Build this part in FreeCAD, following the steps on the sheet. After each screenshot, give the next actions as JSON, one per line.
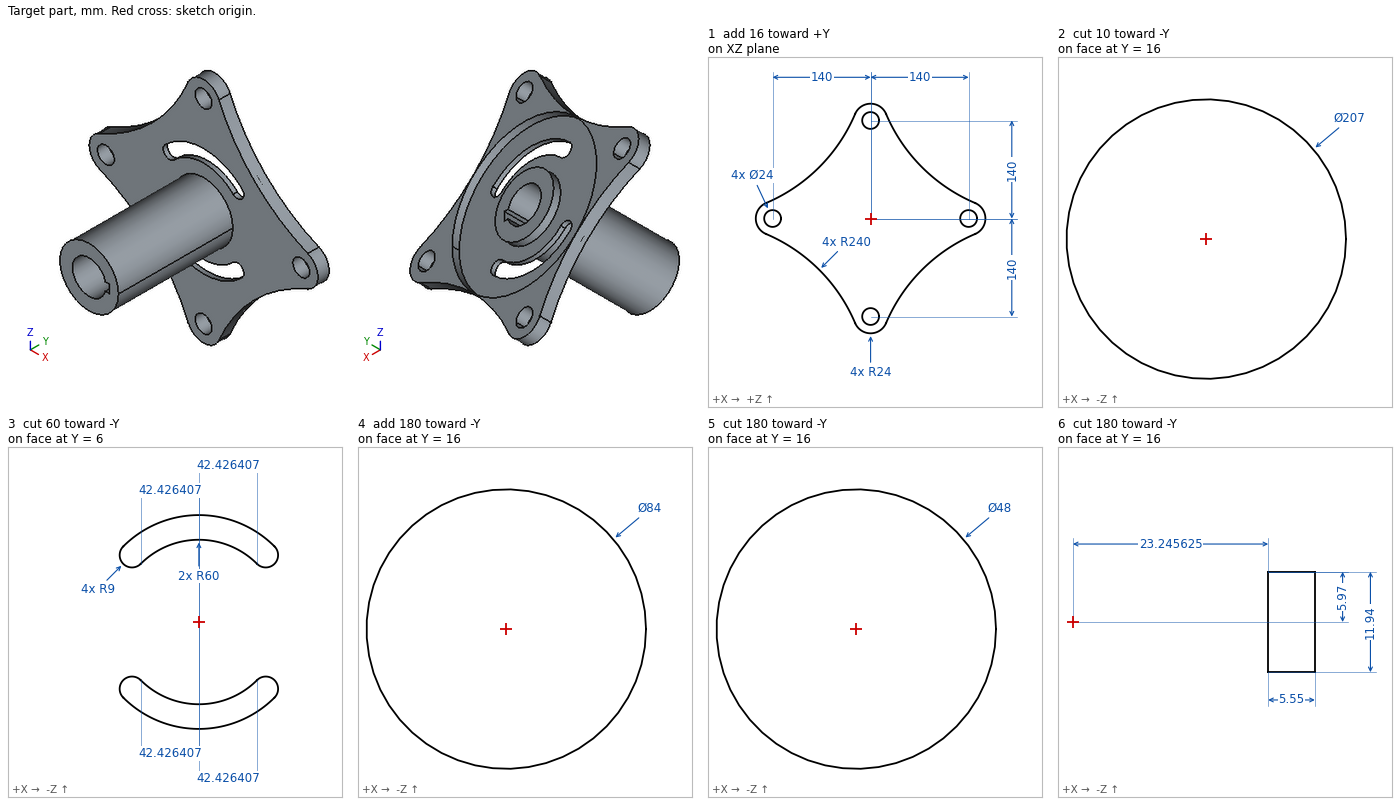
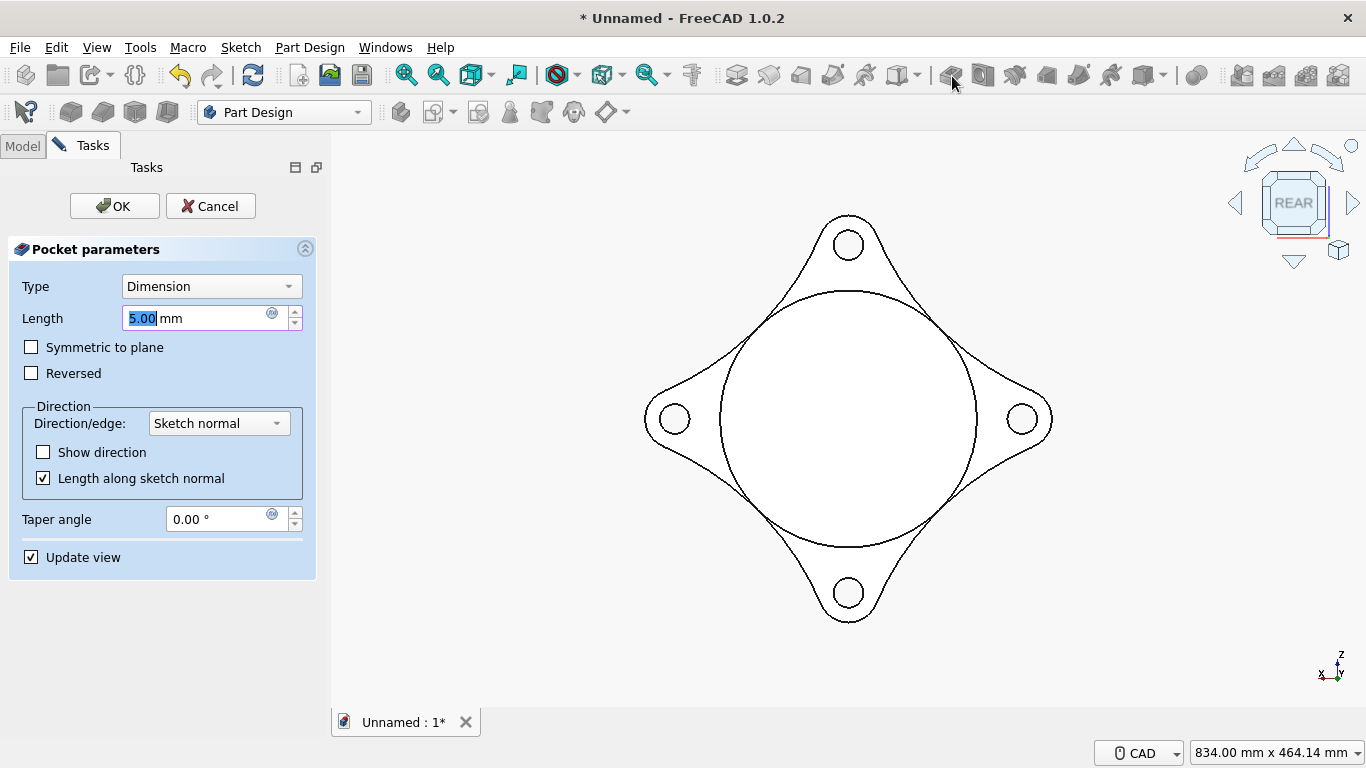
{"action": "type", "text": "10"}
{"action": "key", "text": "Tab"}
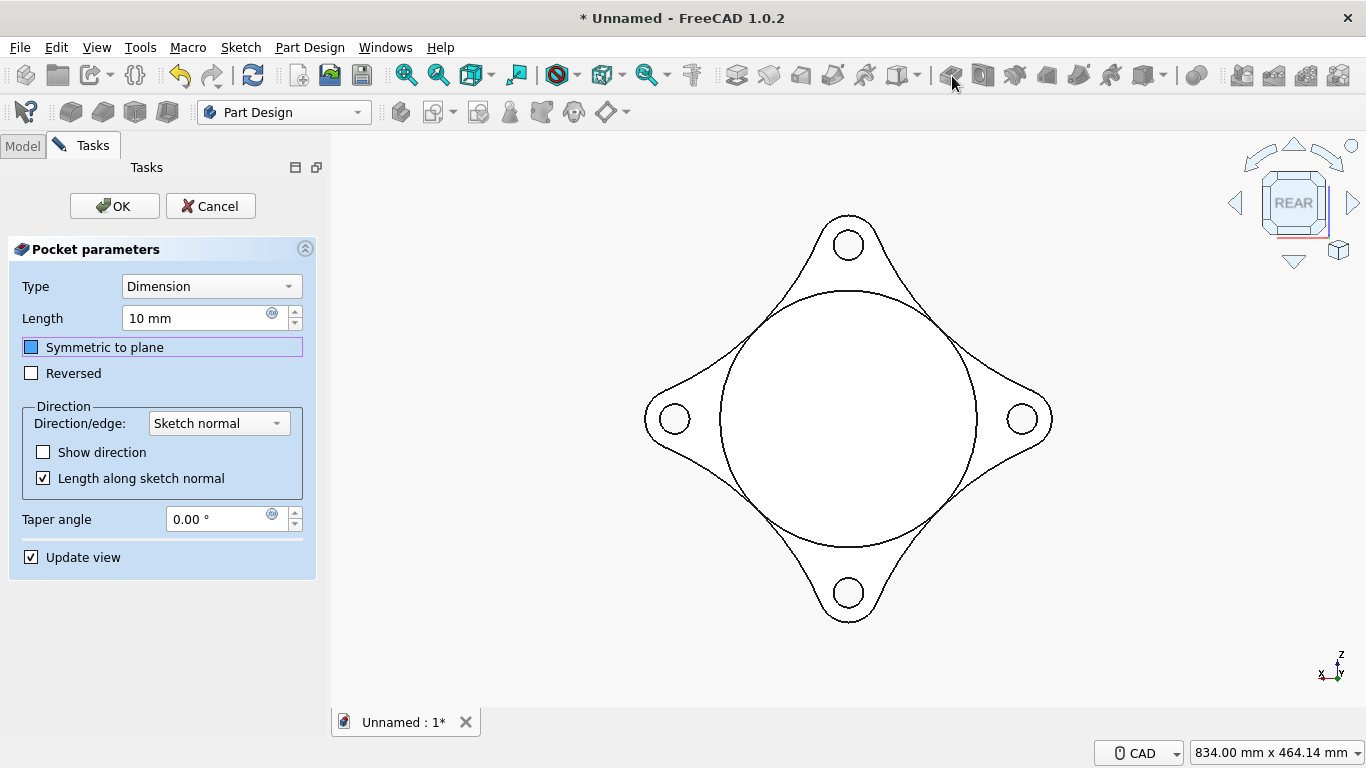
{"action": "left_click", "coordinate": [115, 206]}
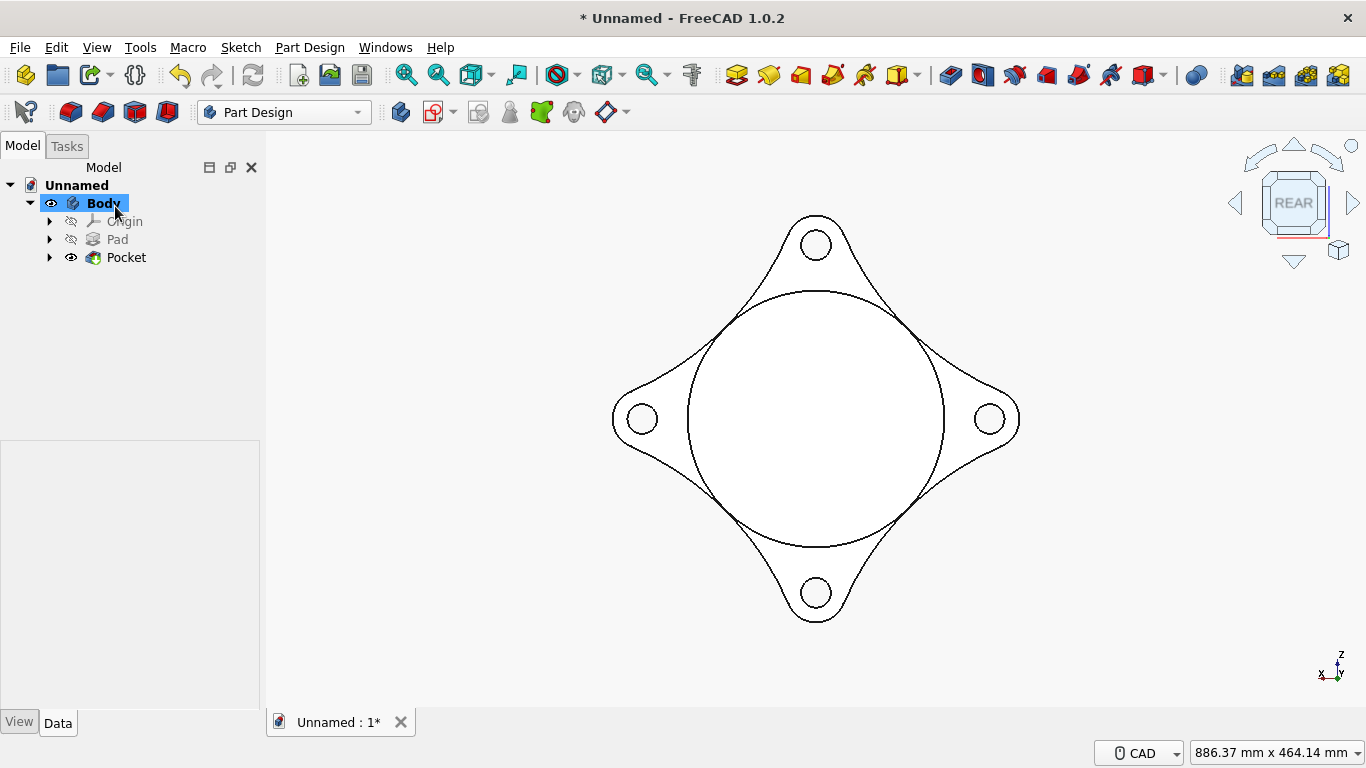
{"action": "left_click", "coordinate": [816, 418]}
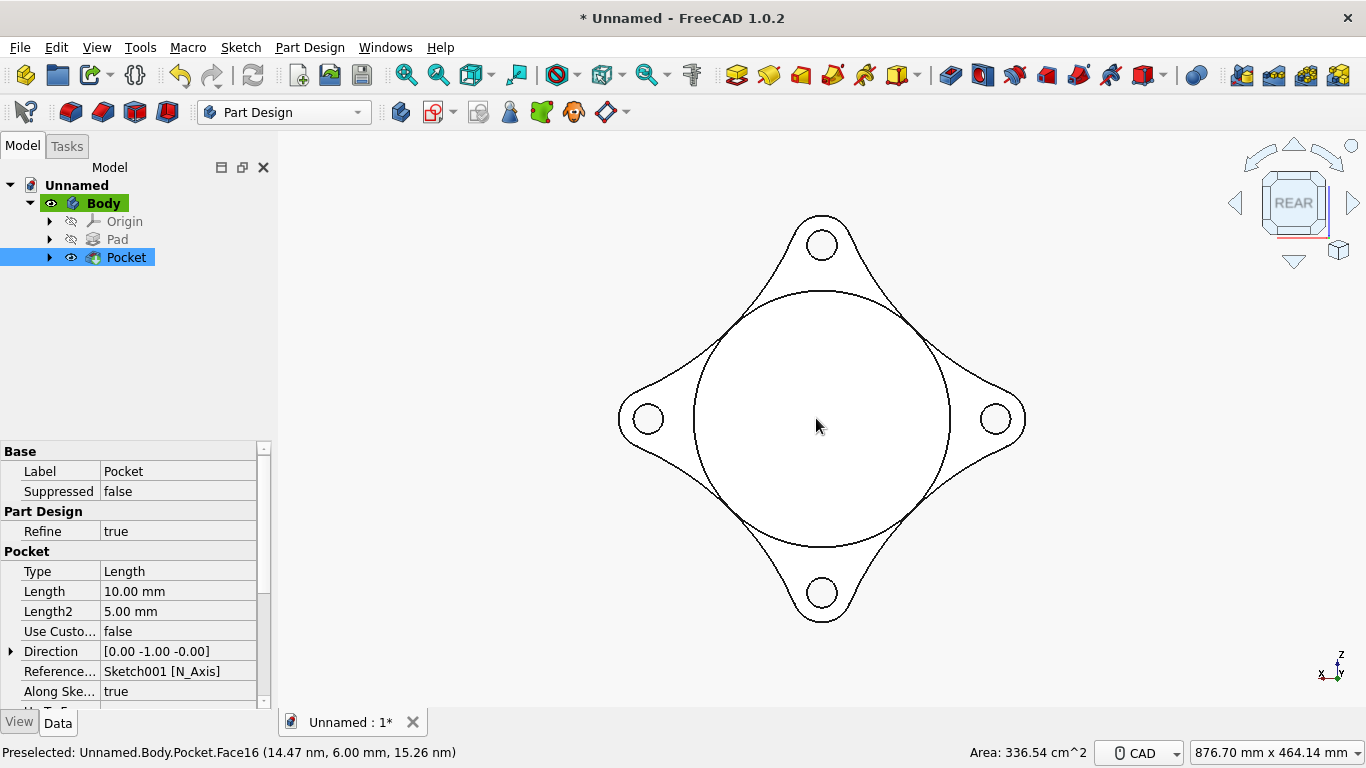
{"action": "left_click", "coordinate": [434, 112]}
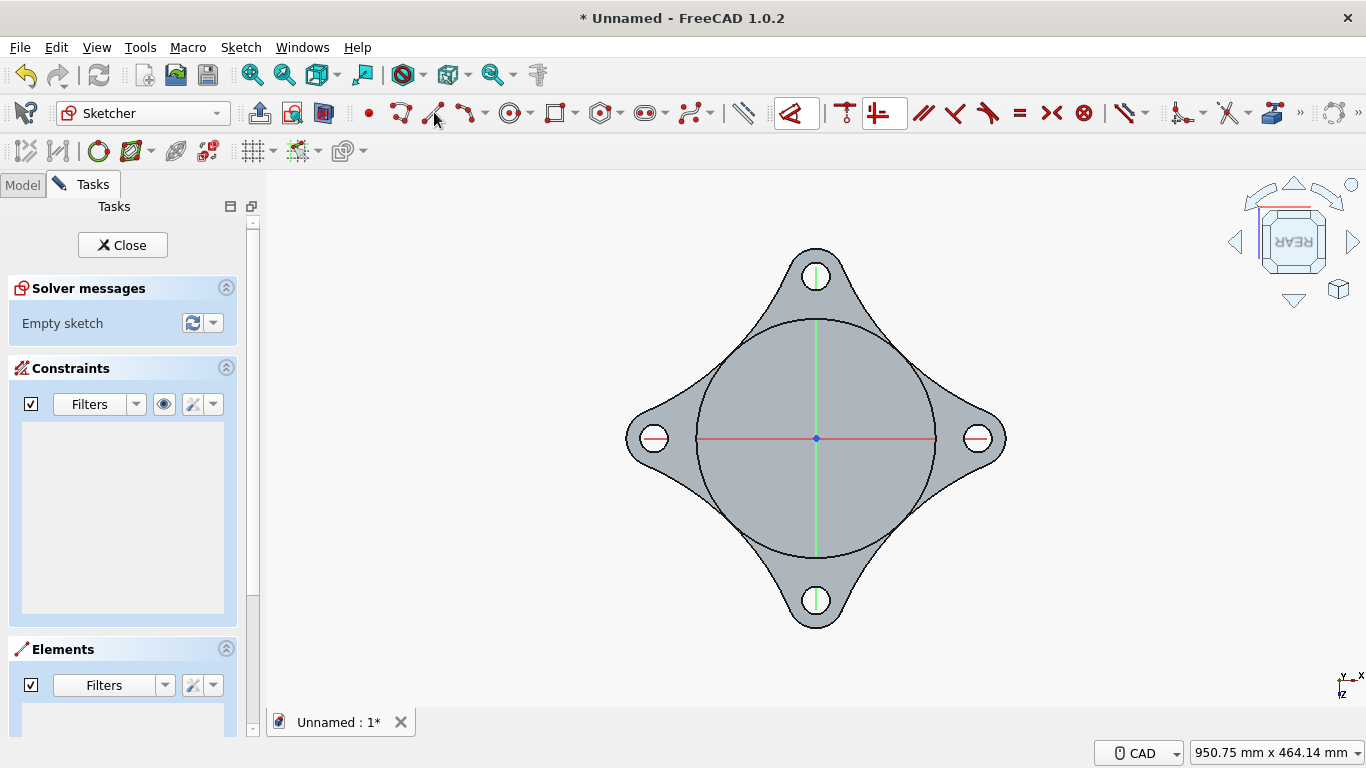
{"action": "left_click", "coordinate": [324, 114]}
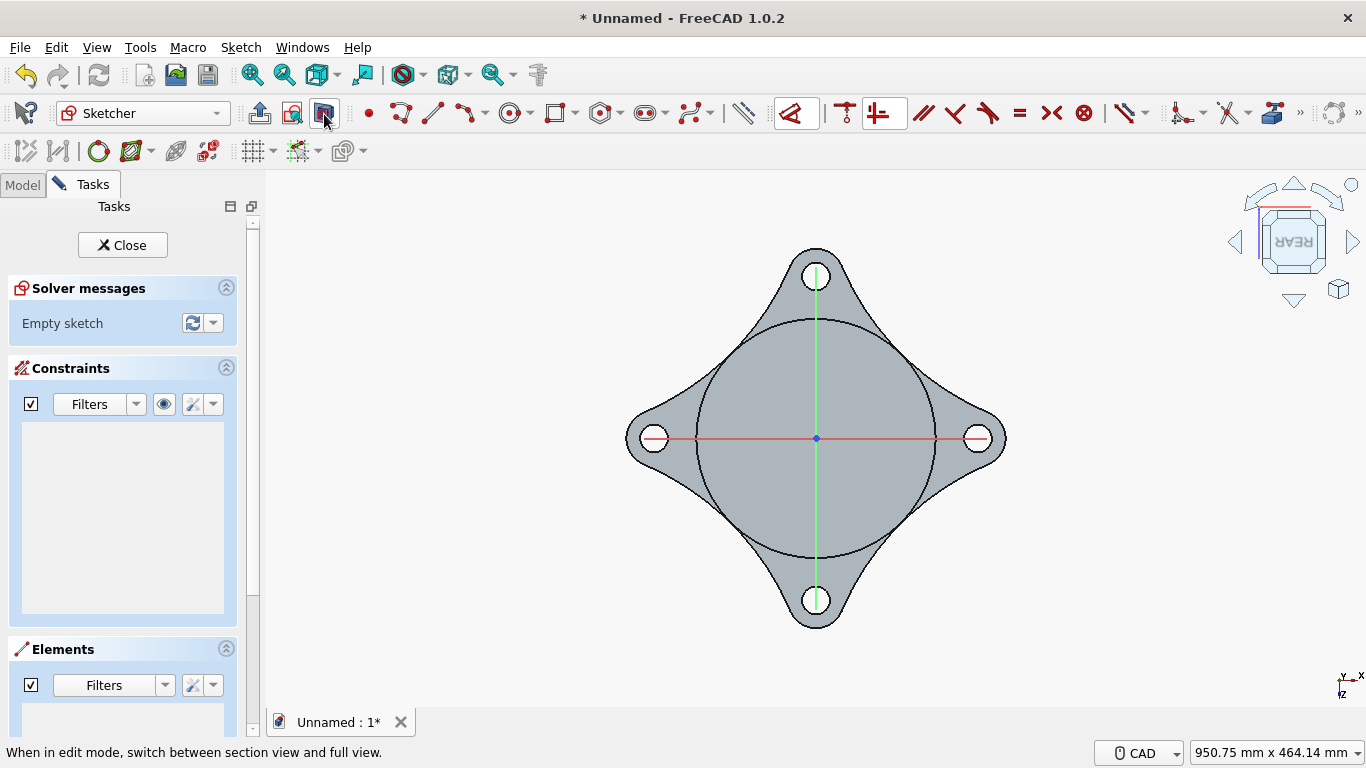
{"action": "scroll", "coordinate": [899, 438], "scroll_direction": "up", "scroll_amount": 3}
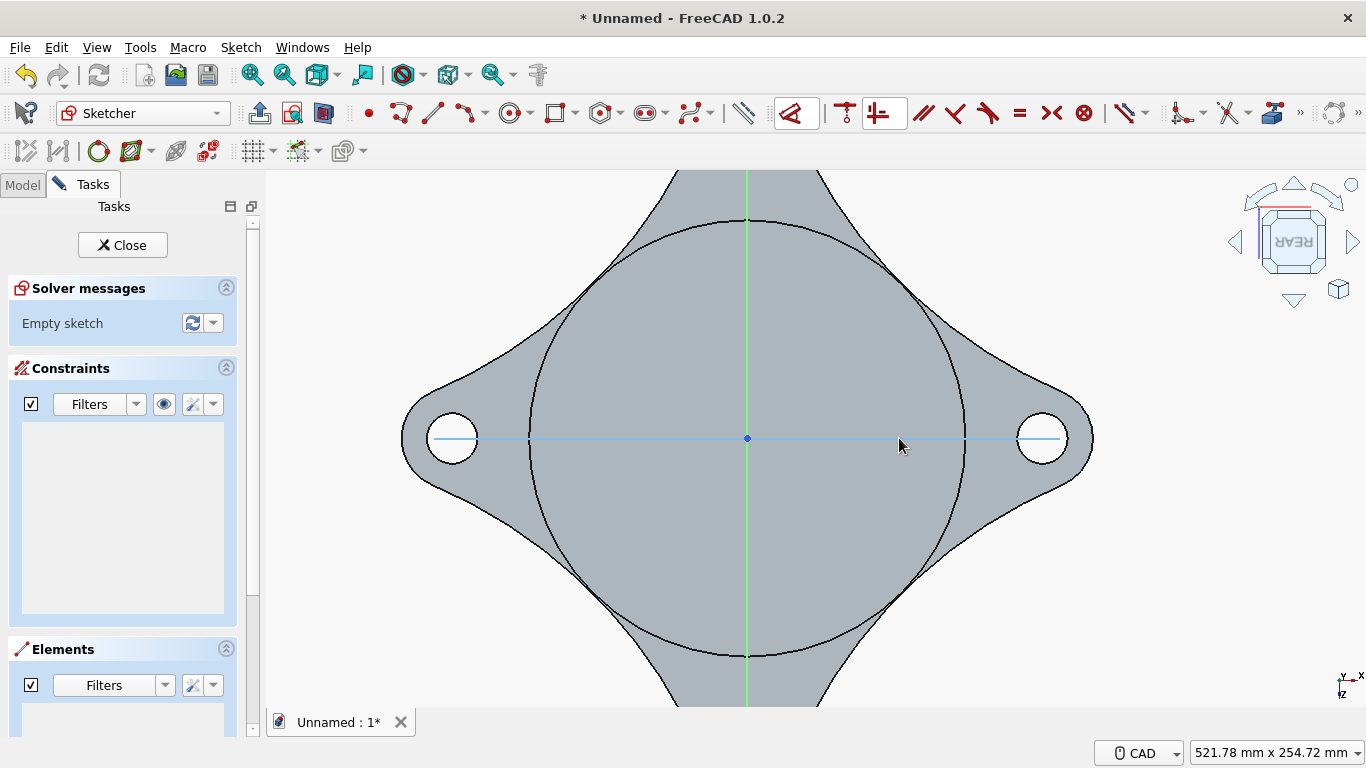
{"action": "left_click", "coordinate": [466, 114]}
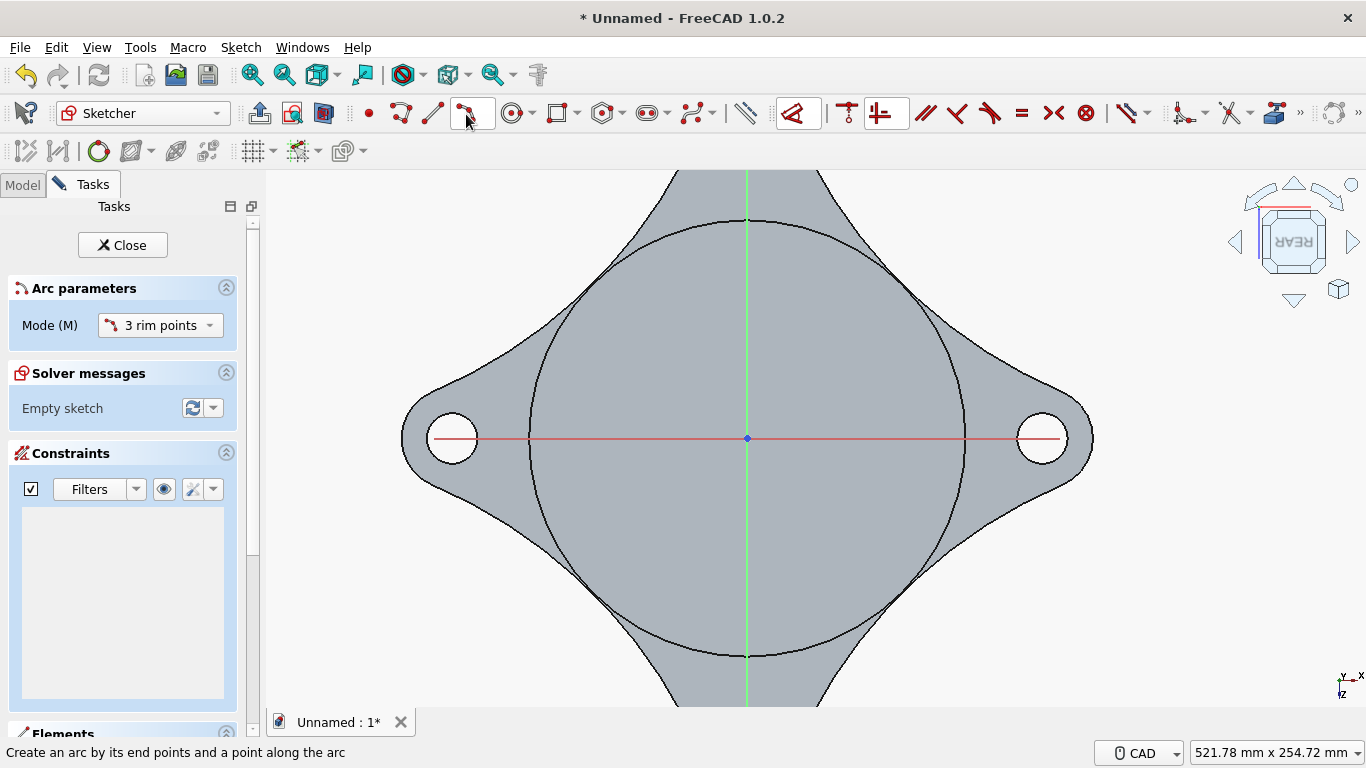
{"action": "left_click", "coordinate": [658, 349]}
{"action": "left_click", "coordinate": [837, 349]}
{"action": "left_click", "coordinate": [767, 314]}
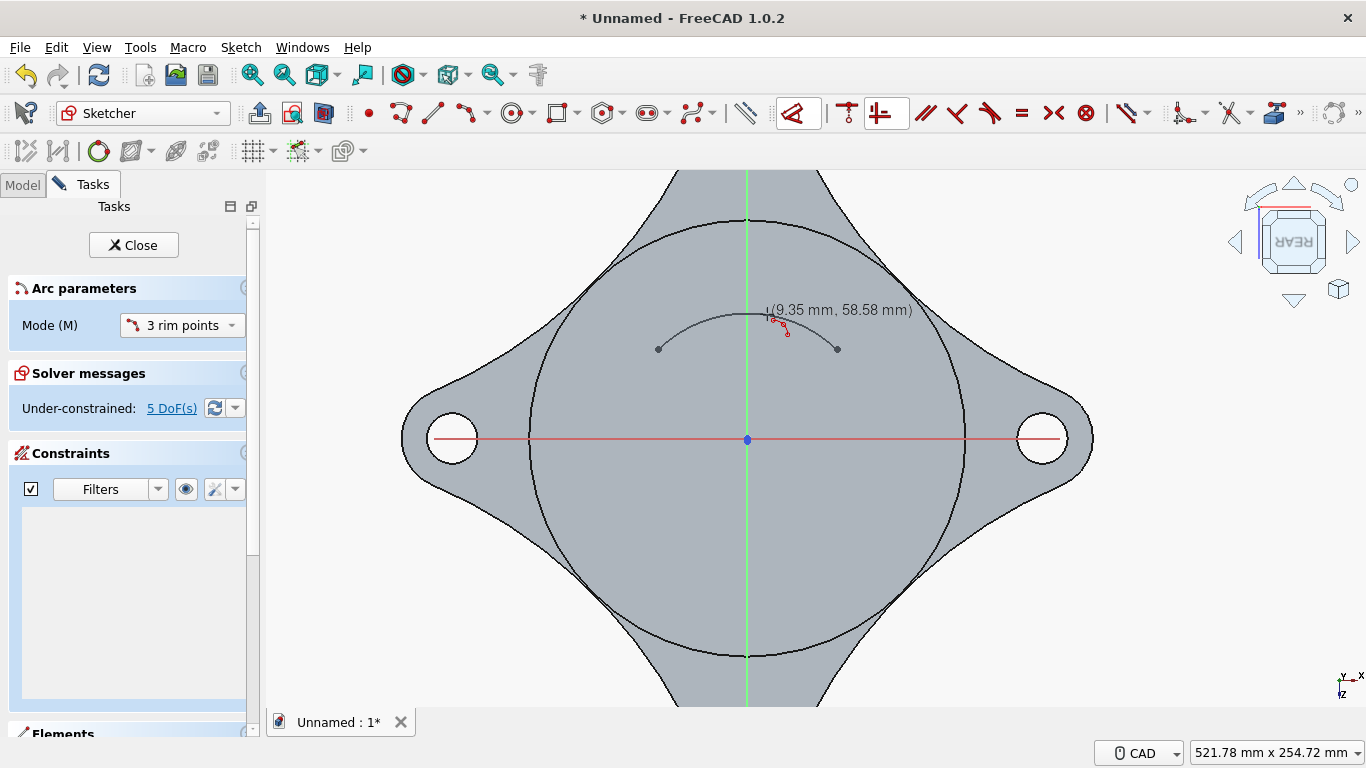
{"action": "left_click", "coordinate": [837, 350]}
{"action": "left_click", "coordinate": [864, 322]}
{"action": "left_click", "coordinate": [864, 349]}